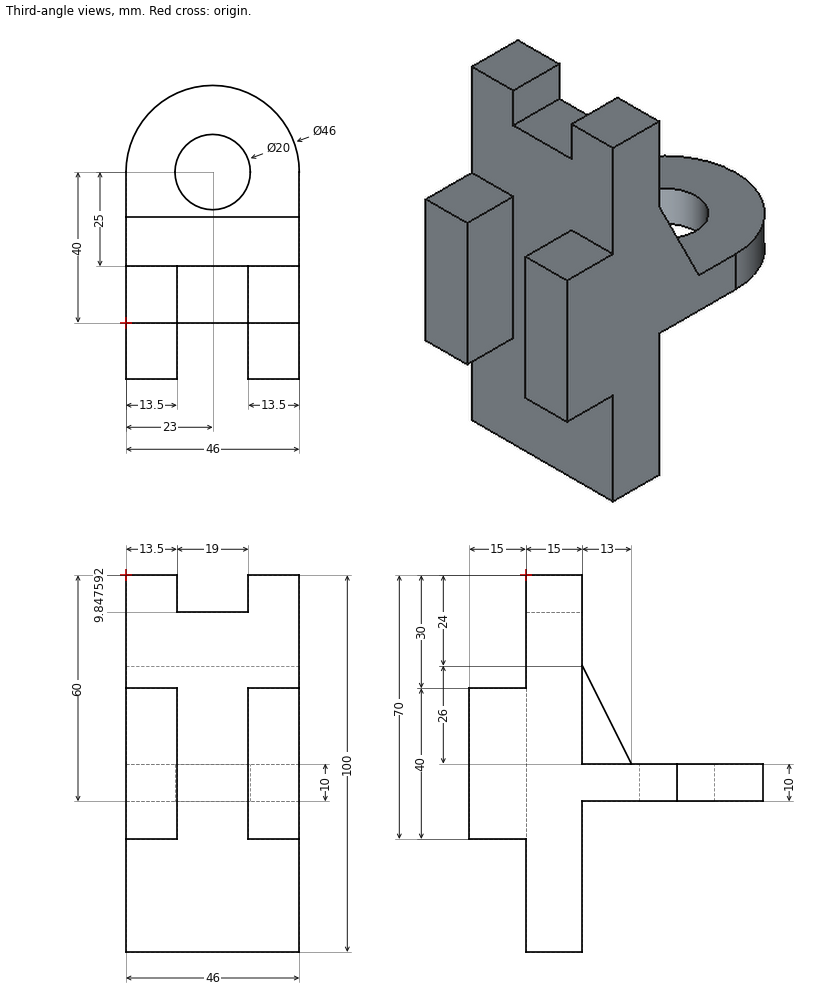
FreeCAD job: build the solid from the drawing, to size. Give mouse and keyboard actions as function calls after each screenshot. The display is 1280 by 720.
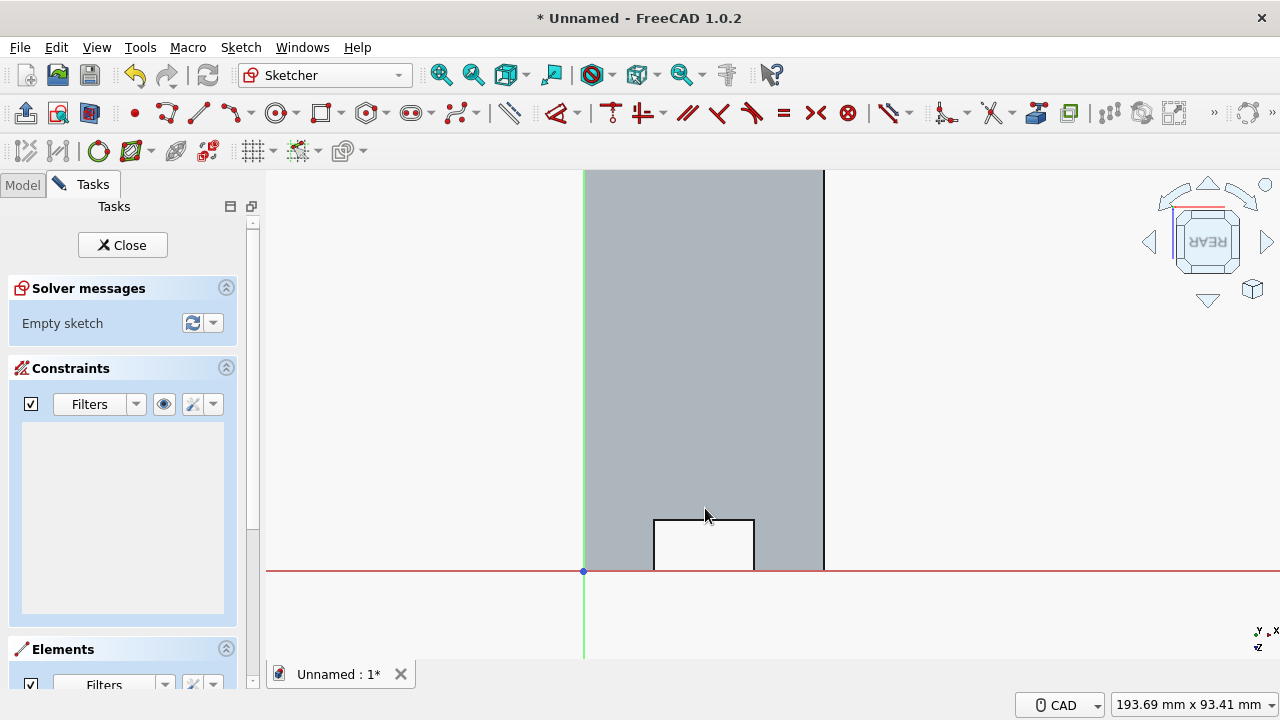
key(g)
key(r)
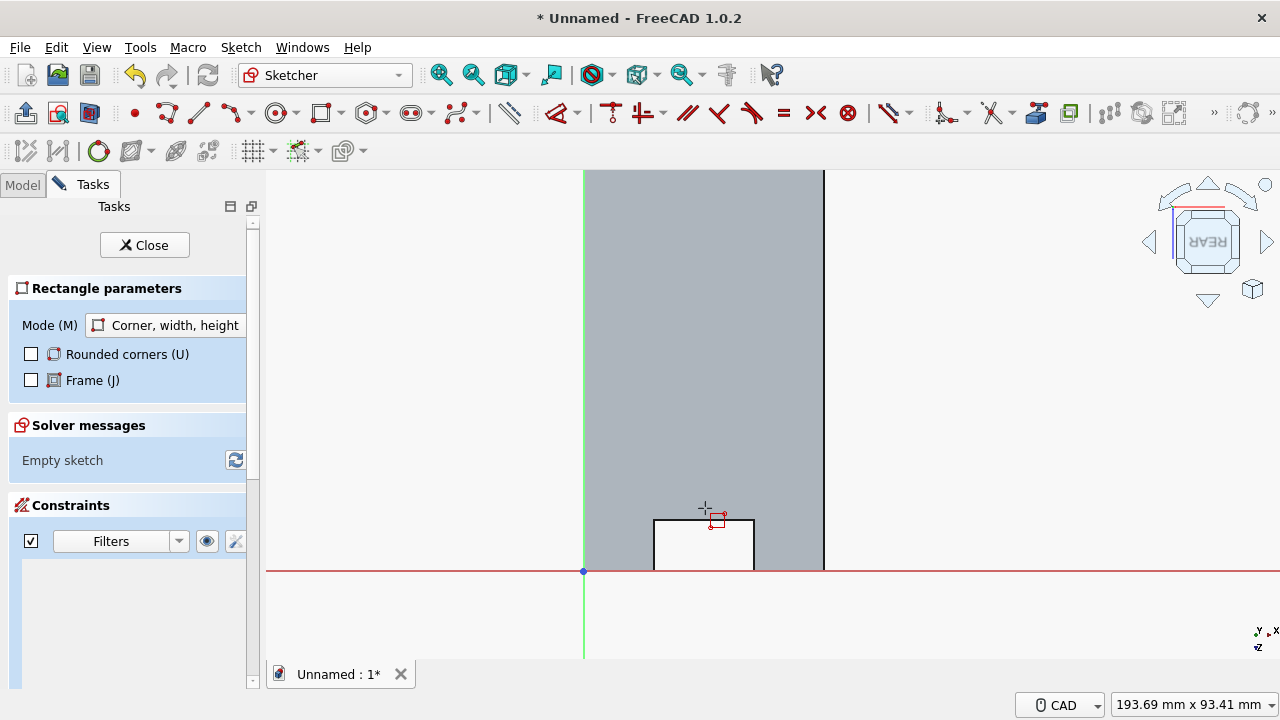
click(584, 257)
move(824, 310)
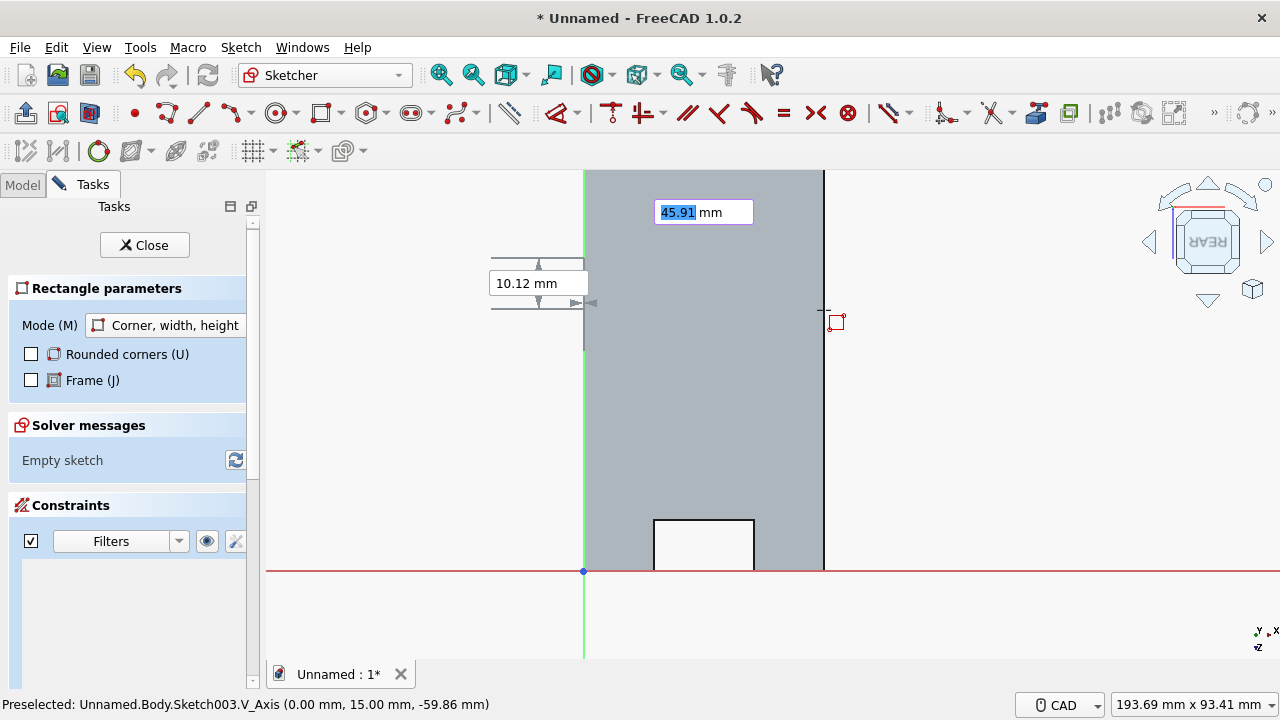
text(46)
key(Tab)
text(10)
key(Return)
key(Escape)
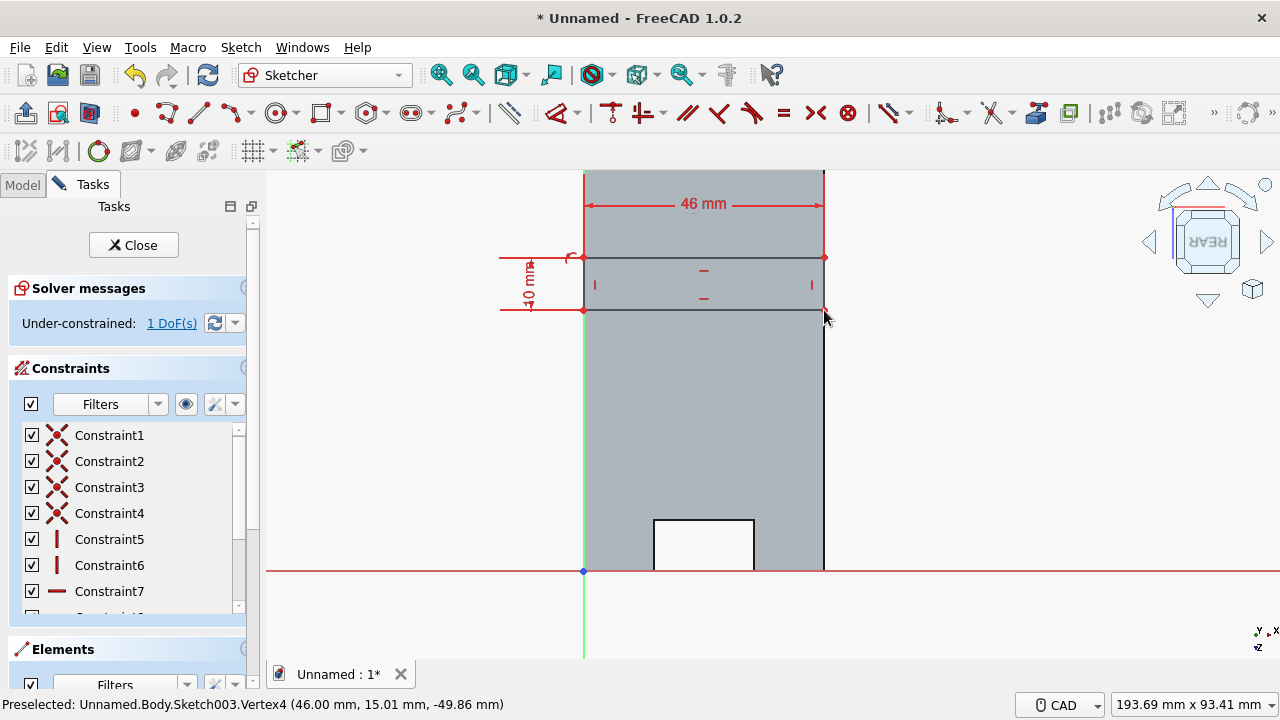
click(556, 114)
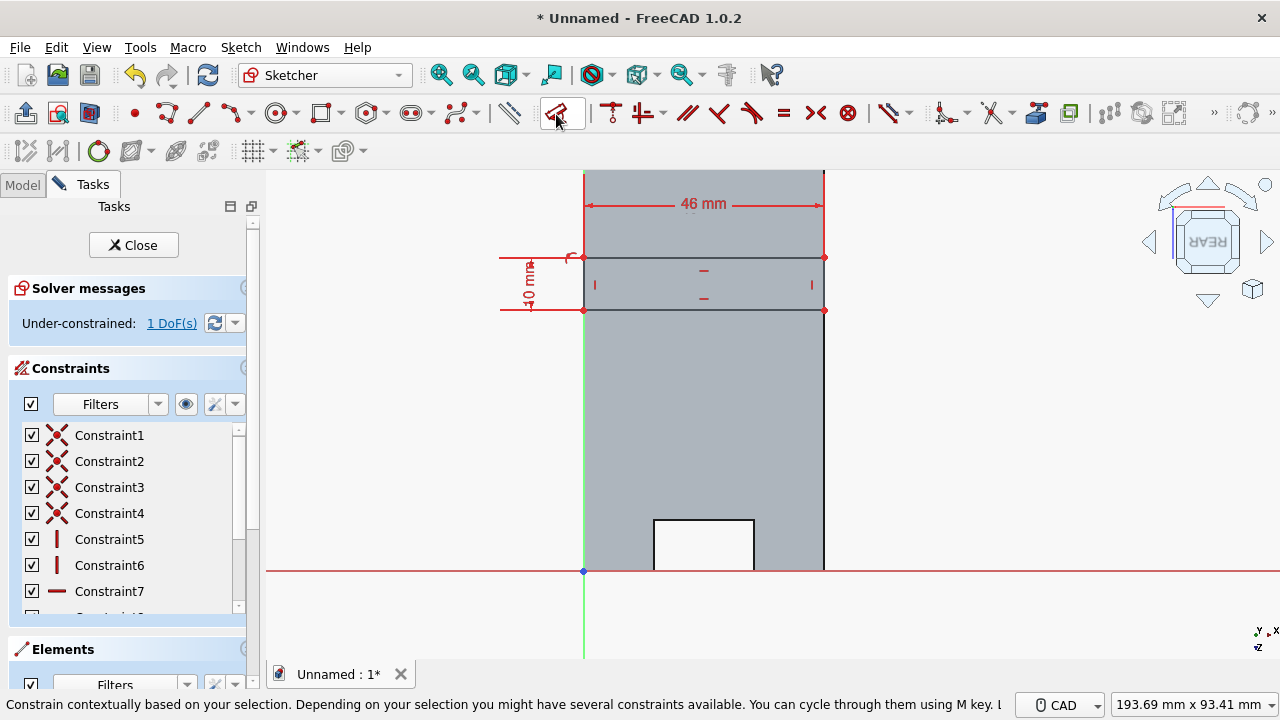
click(584, 258)
click(550, 415)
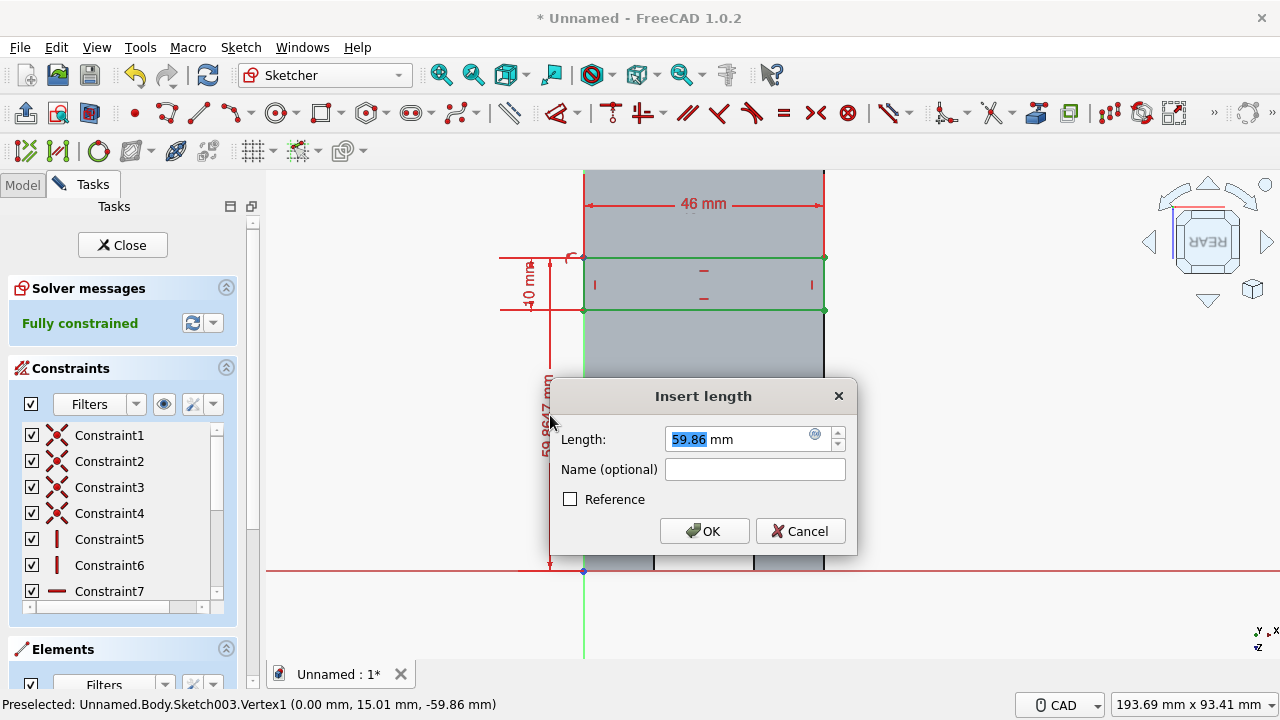
text(60)
key(Return)
key(Escape)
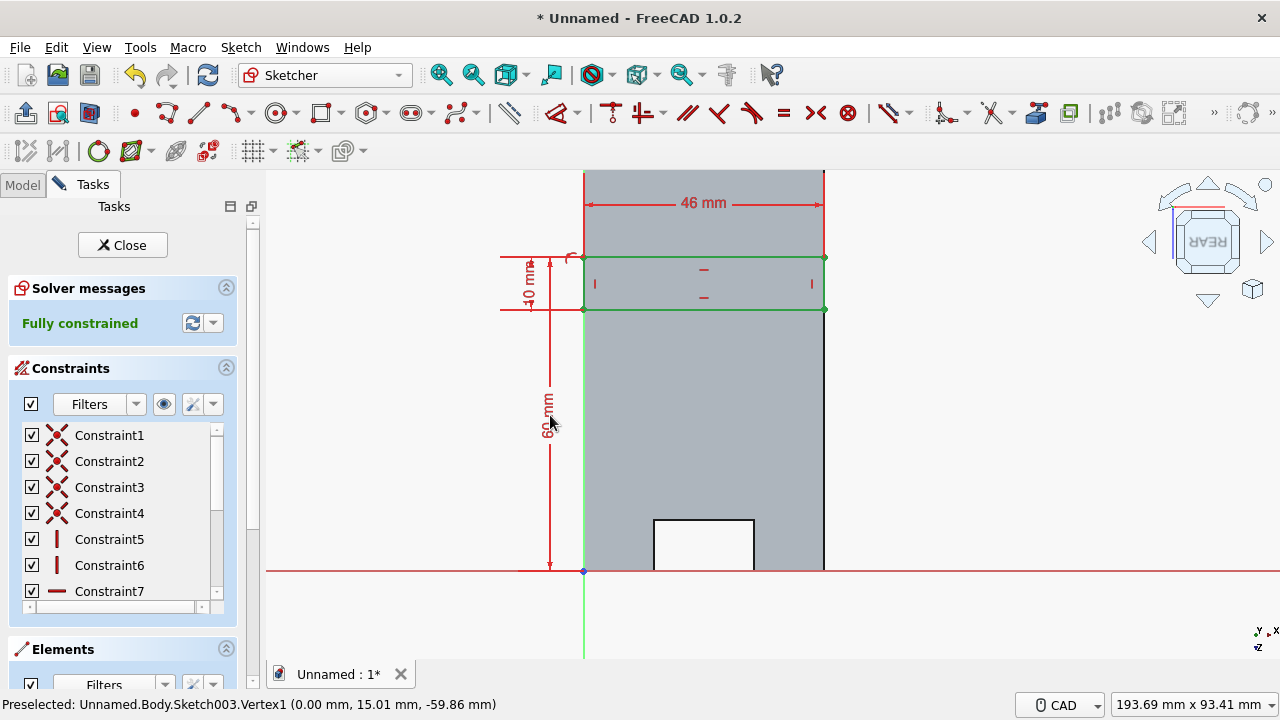
click(123, 245)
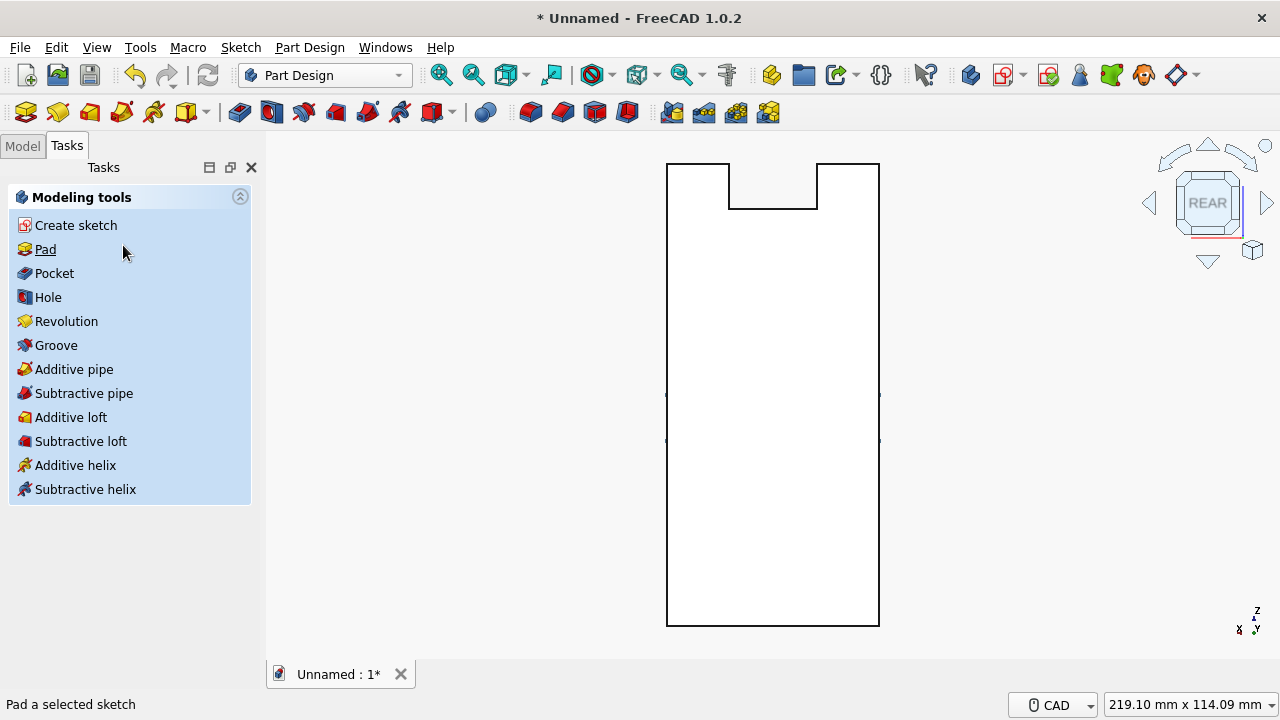
click(26, 112)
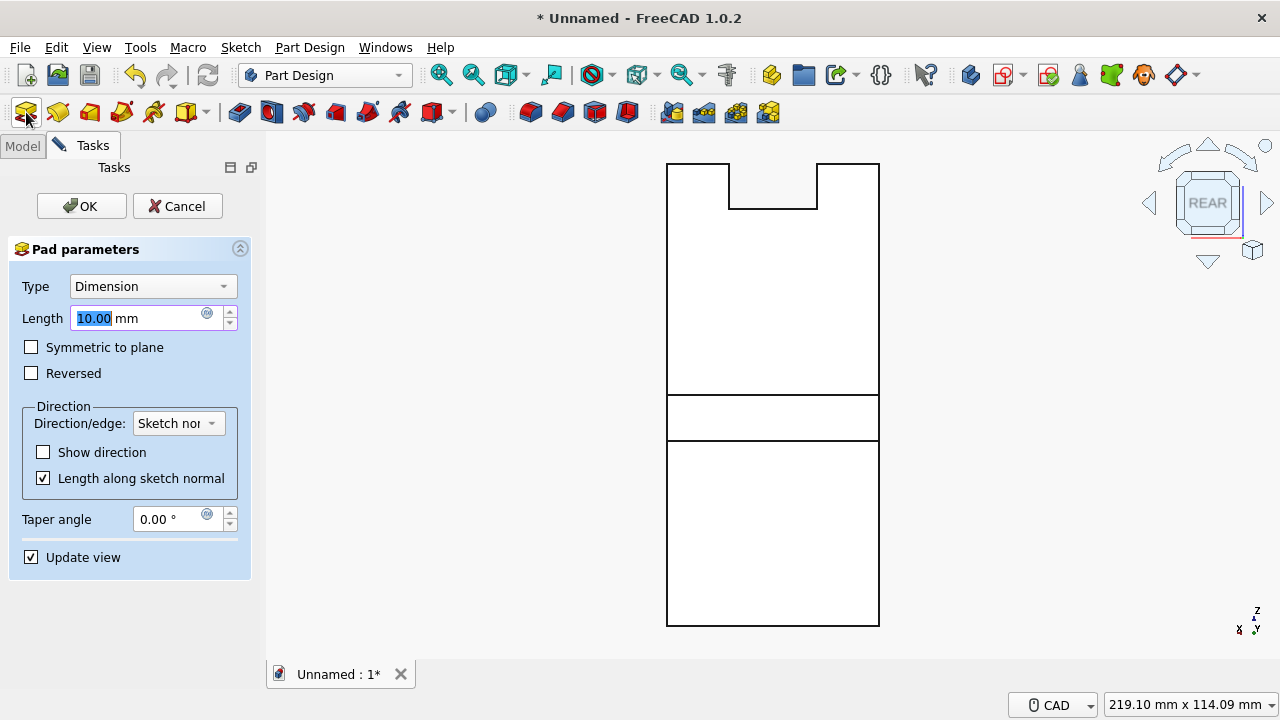
text(25)
key(Tab)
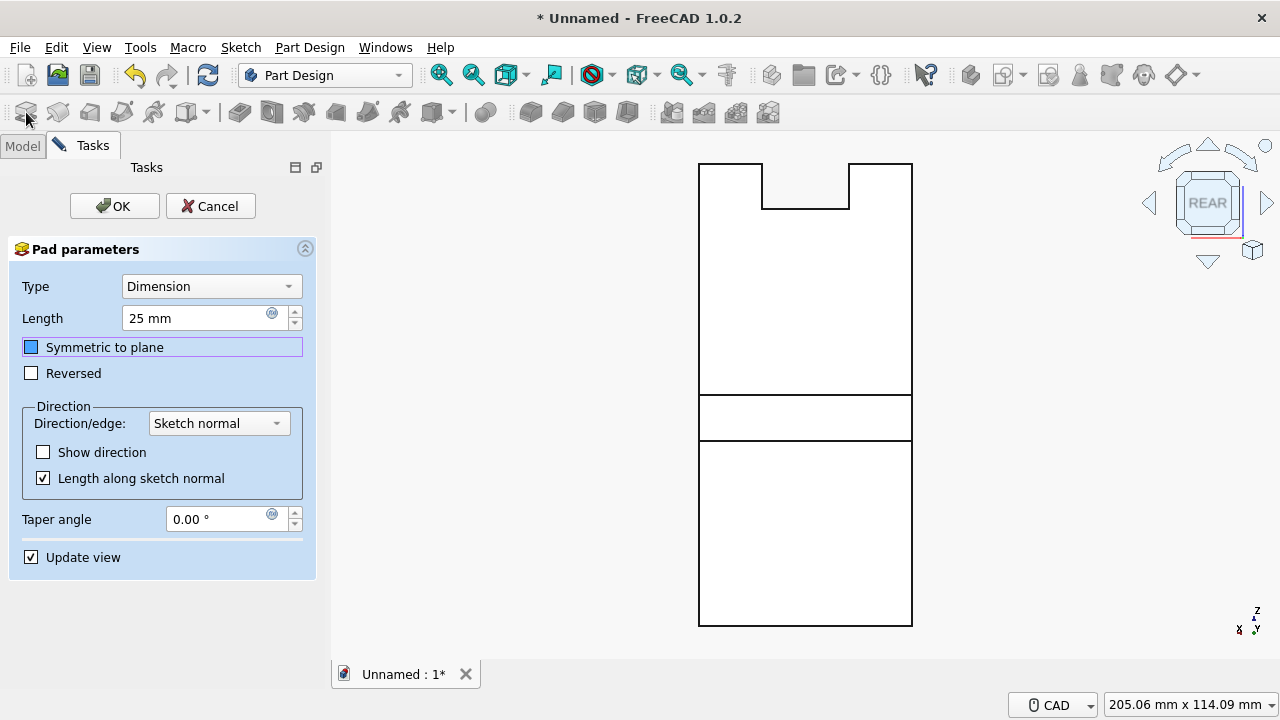
click(115, 206)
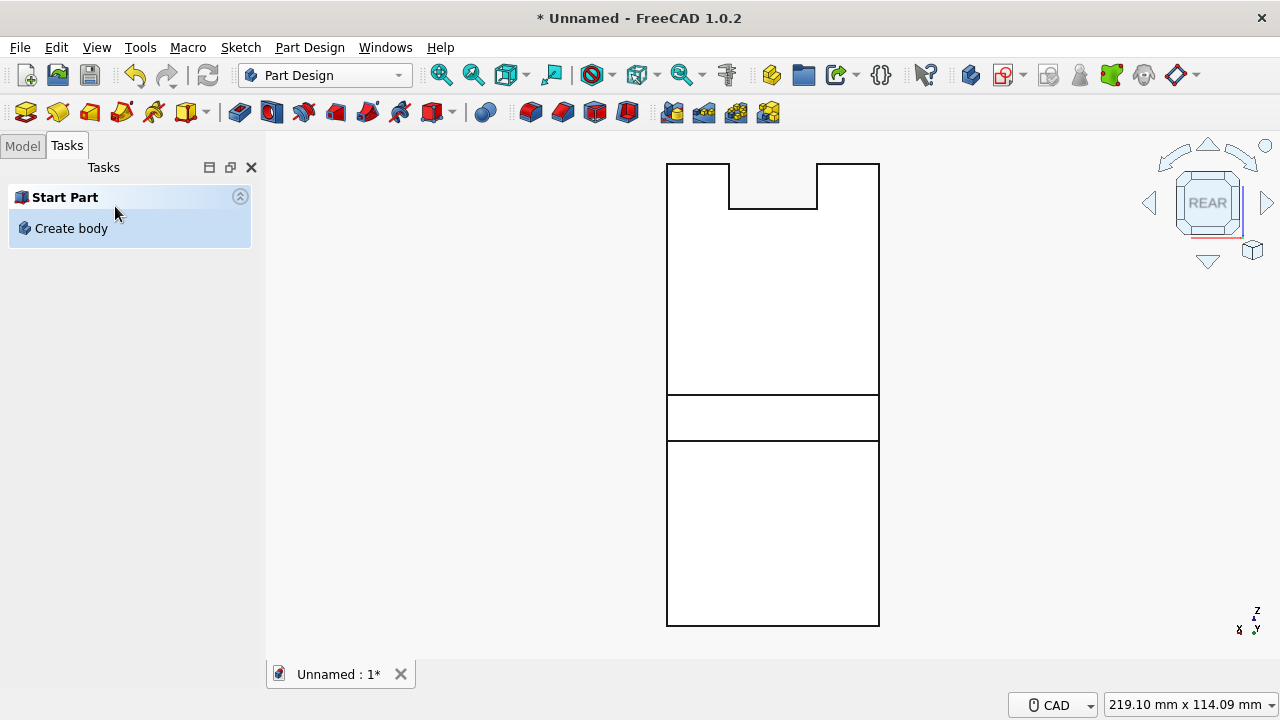
key(0)